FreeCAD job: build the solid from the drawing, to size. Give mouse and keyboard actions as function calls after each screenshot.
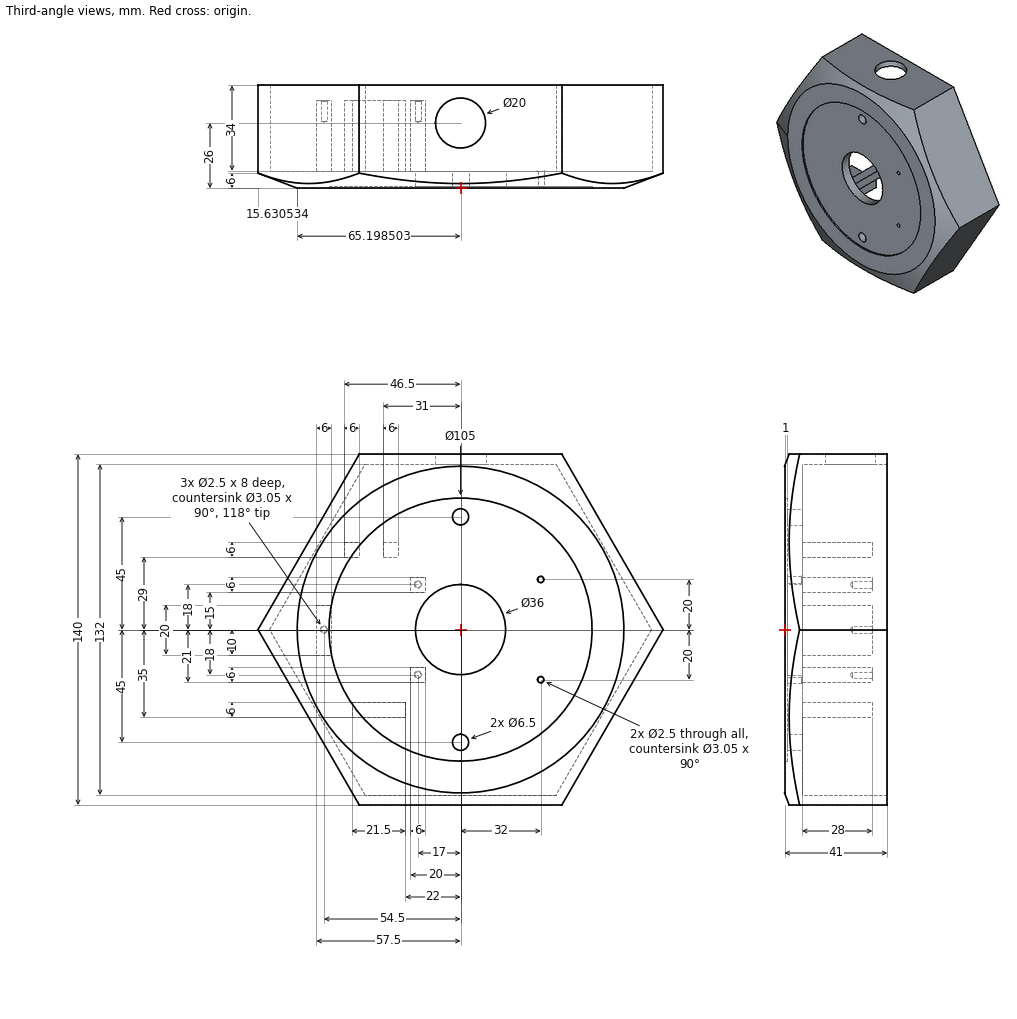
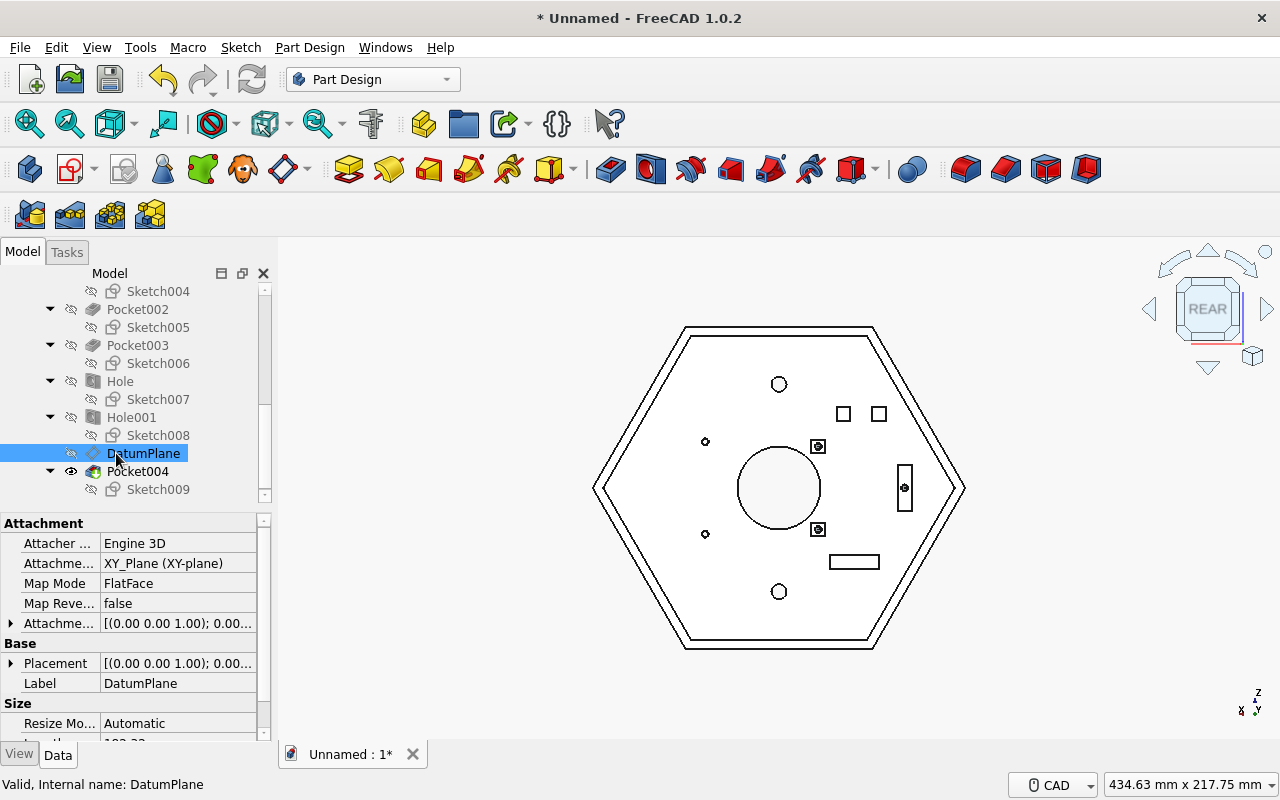
key(0)